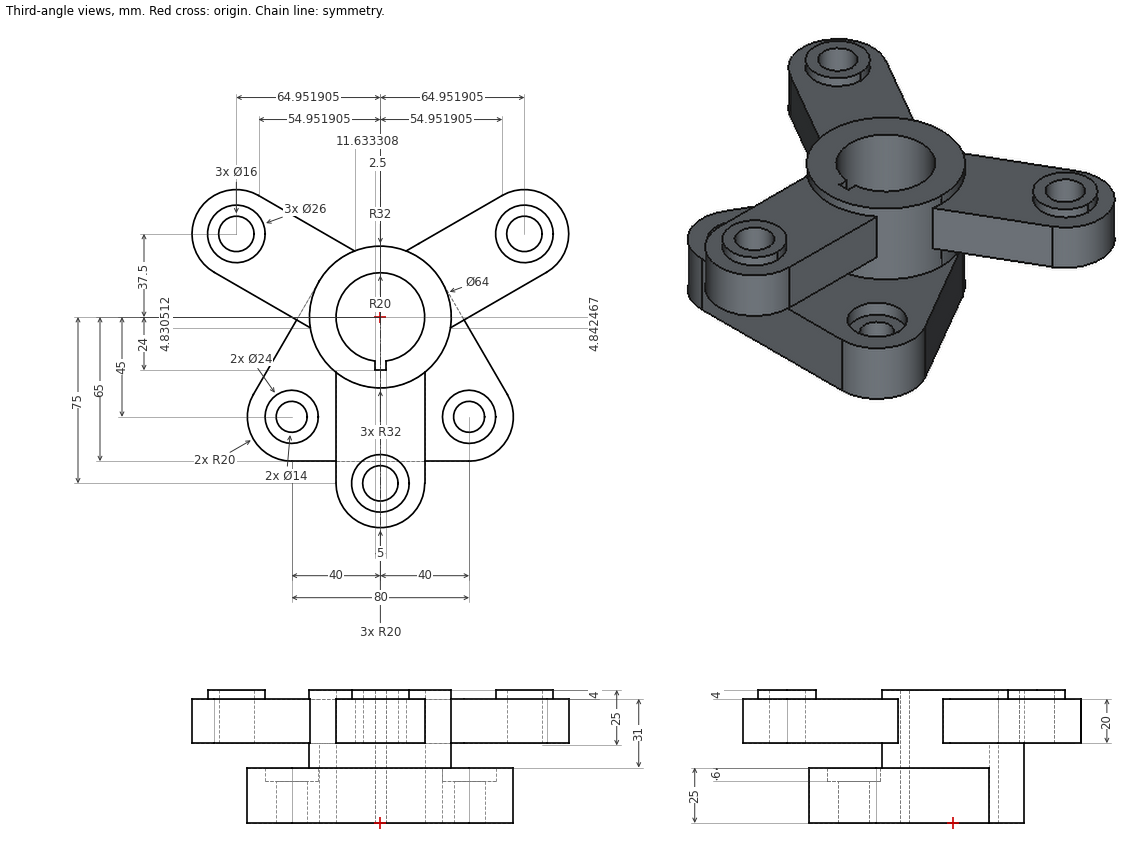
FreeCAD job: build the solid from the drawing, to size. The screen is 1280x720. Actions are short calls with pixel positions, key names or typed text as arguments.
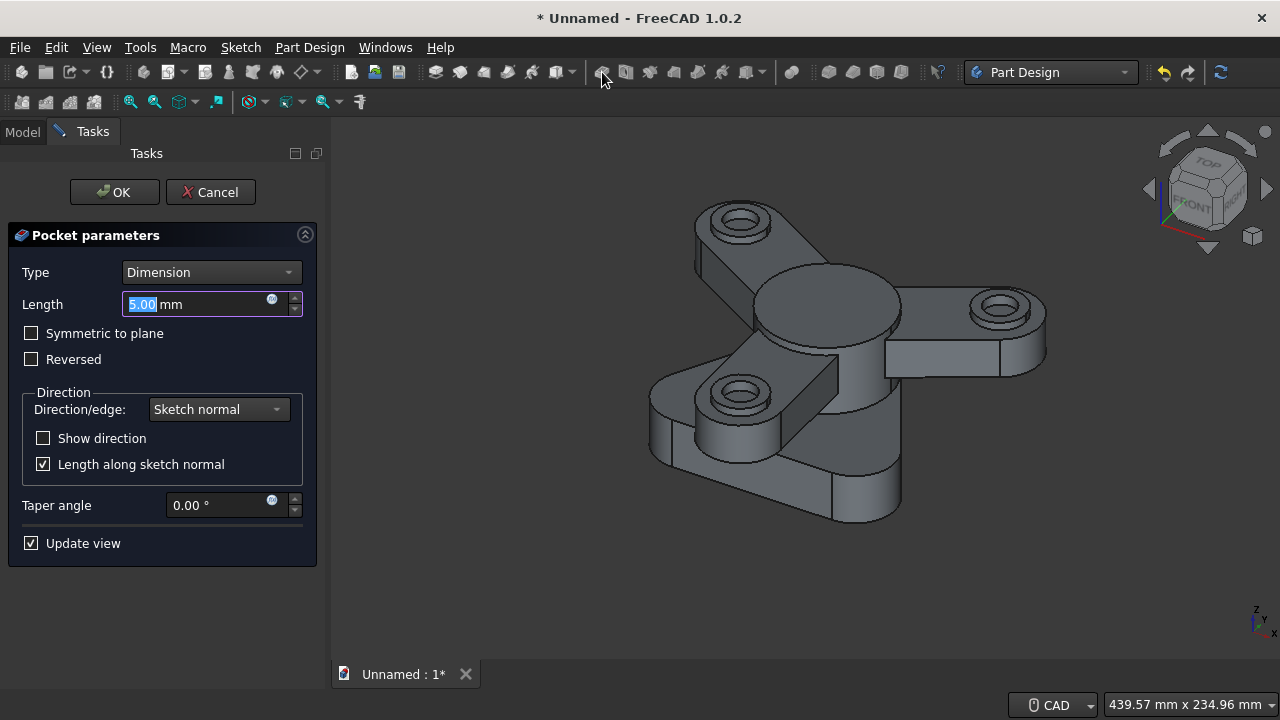
text(25)
key(Tab)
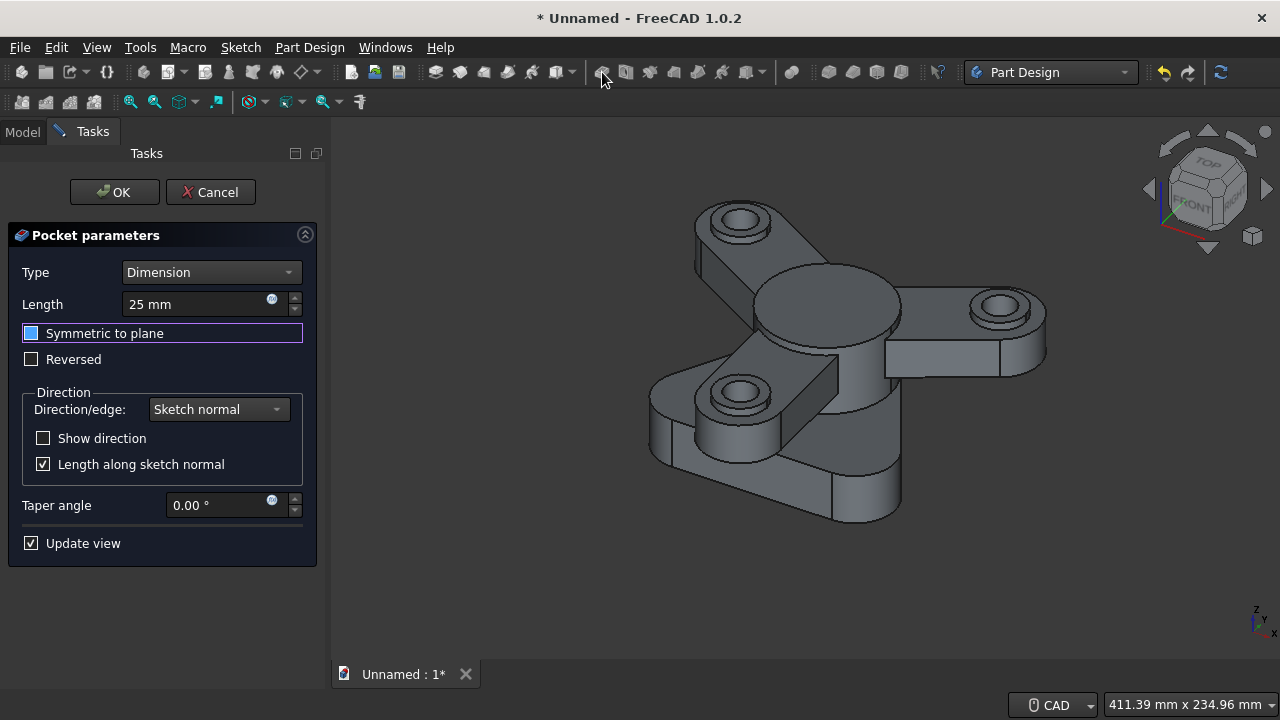
click(115, 192)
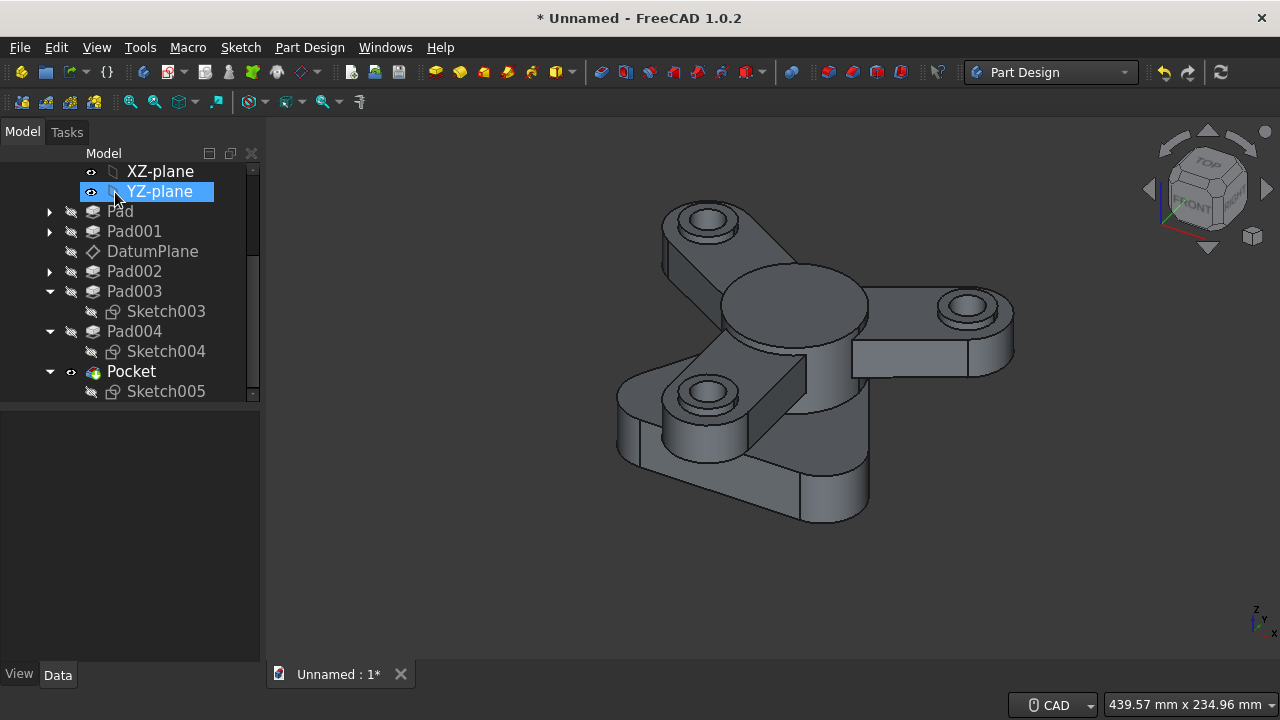
click(795, 305)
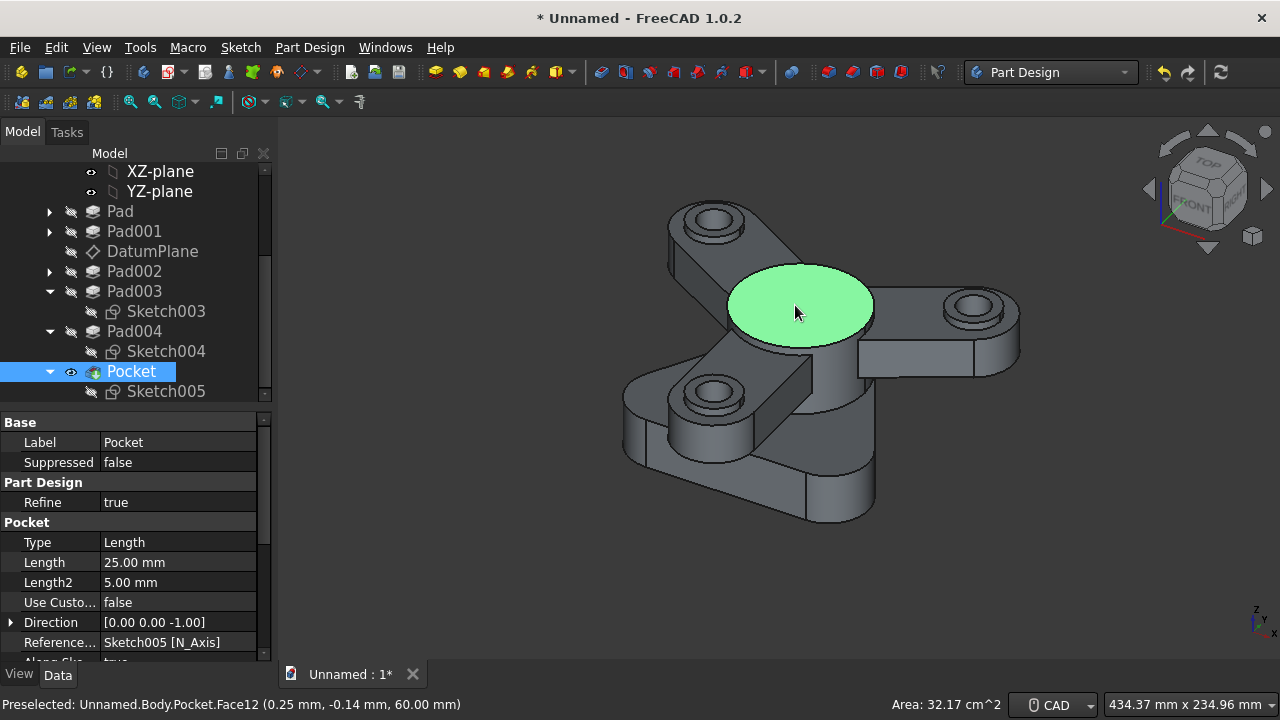
click(168, 72)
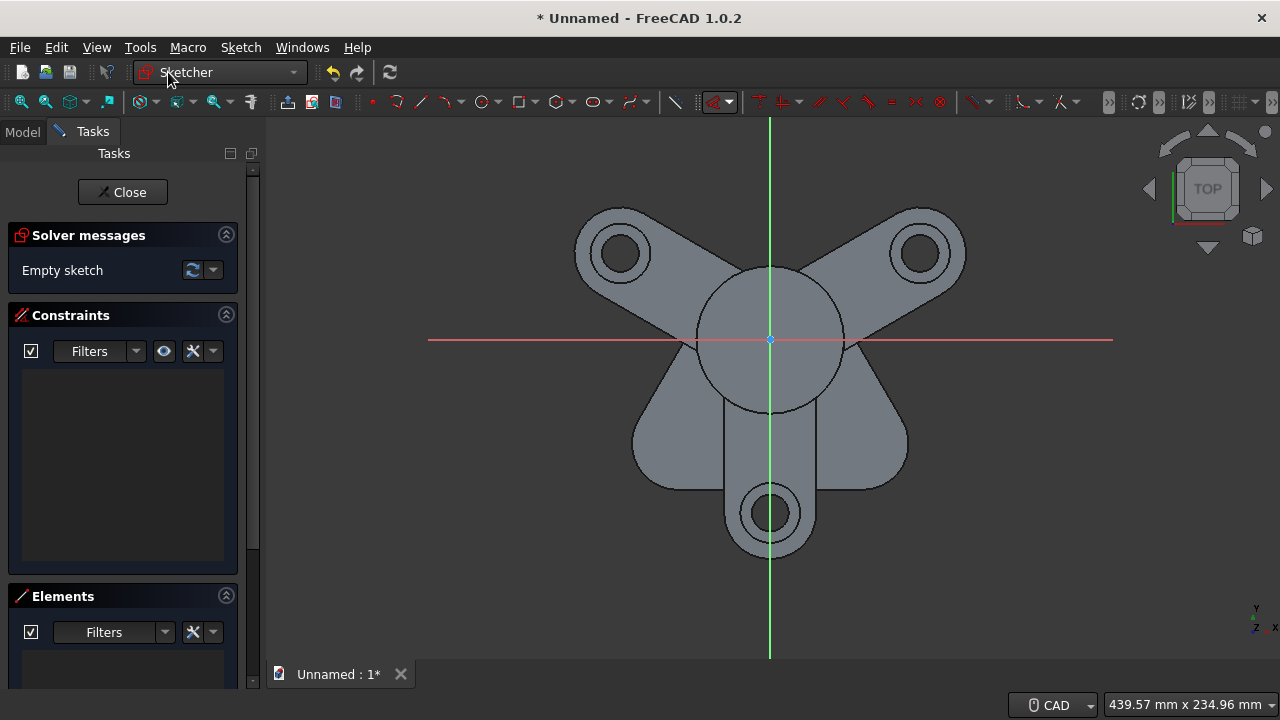
scroll(799, 326, up, 6)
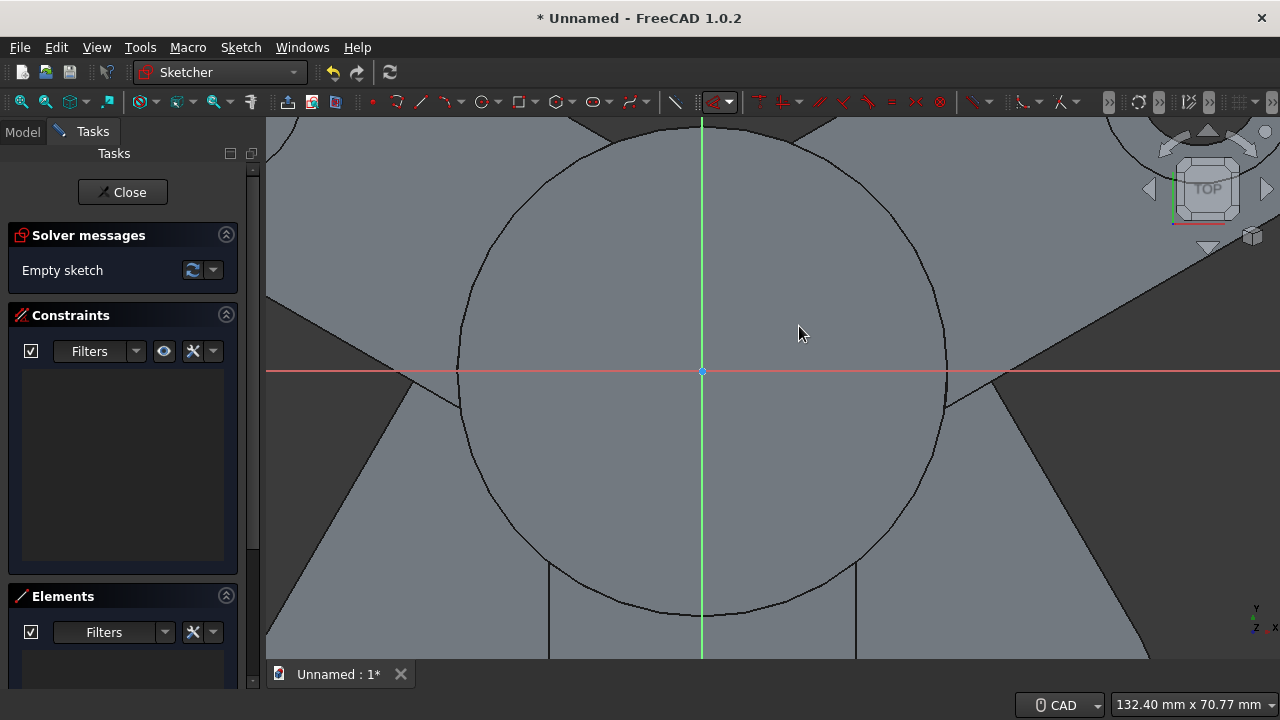
key(g)
key(m)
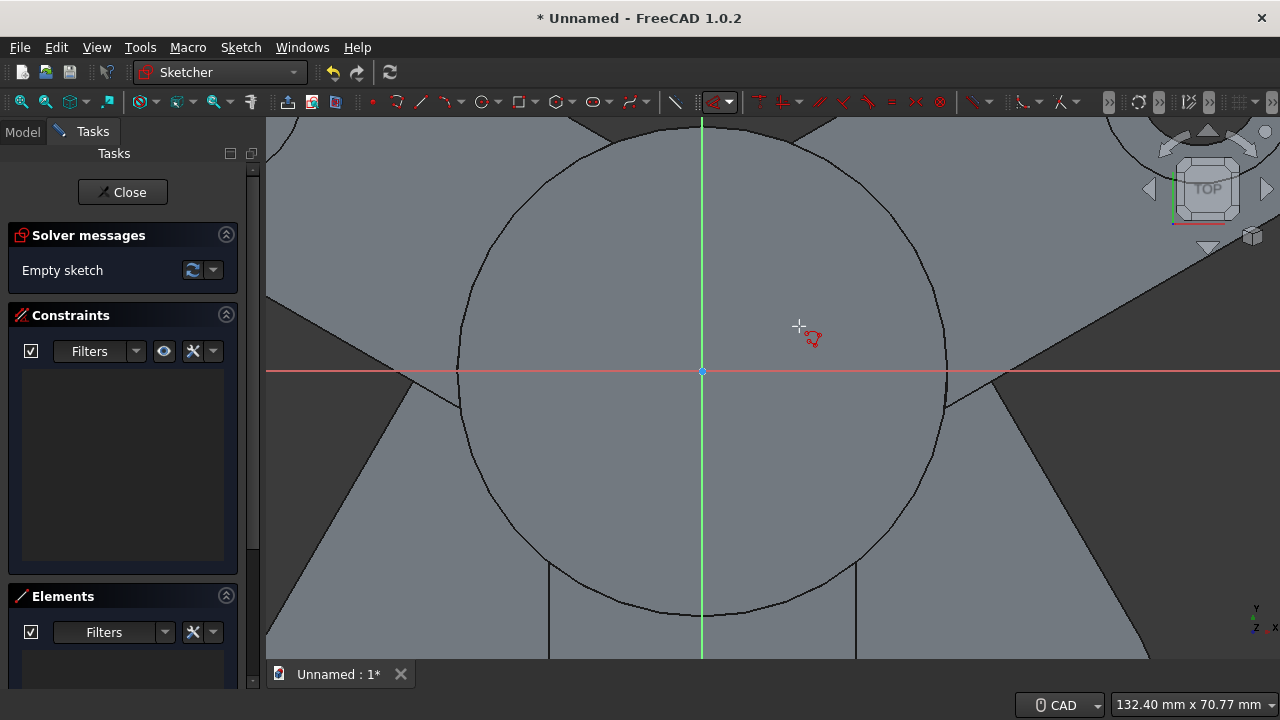
click(683, 523)
click(683, 555)
click(722, 555)
click(722, 523)
right_click(722, 523)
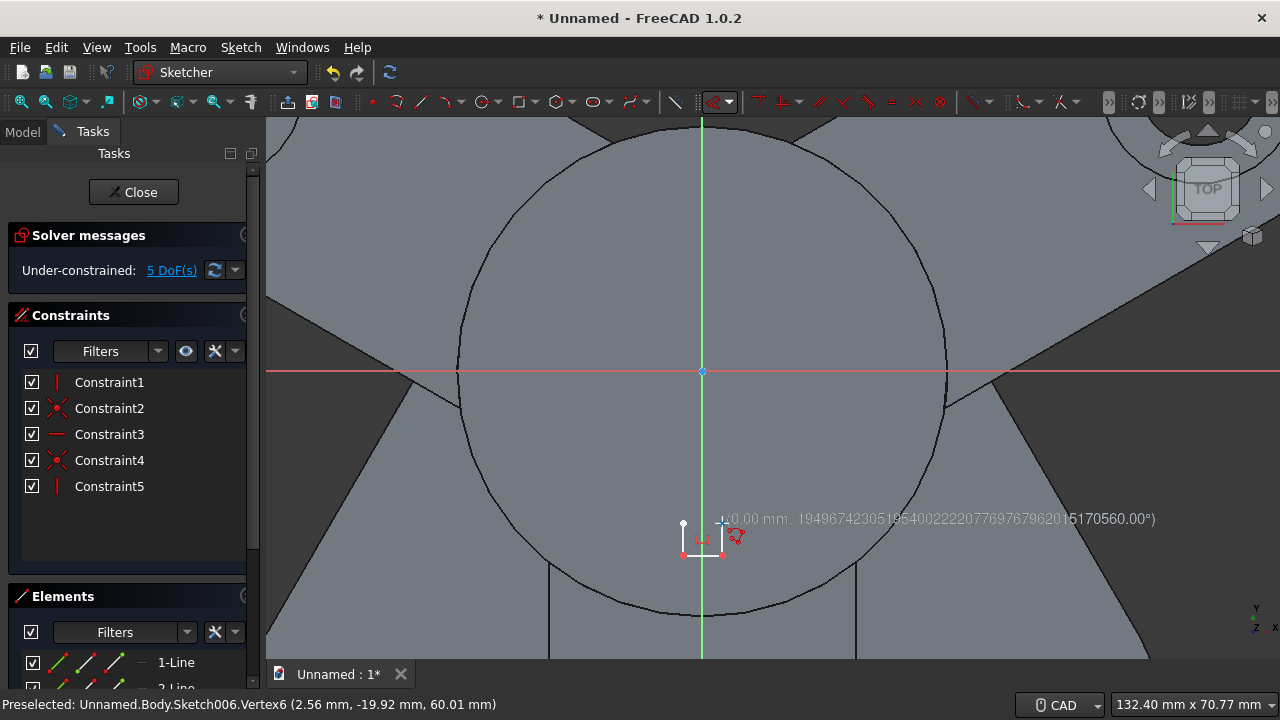
key(g)
key(3)
key(a)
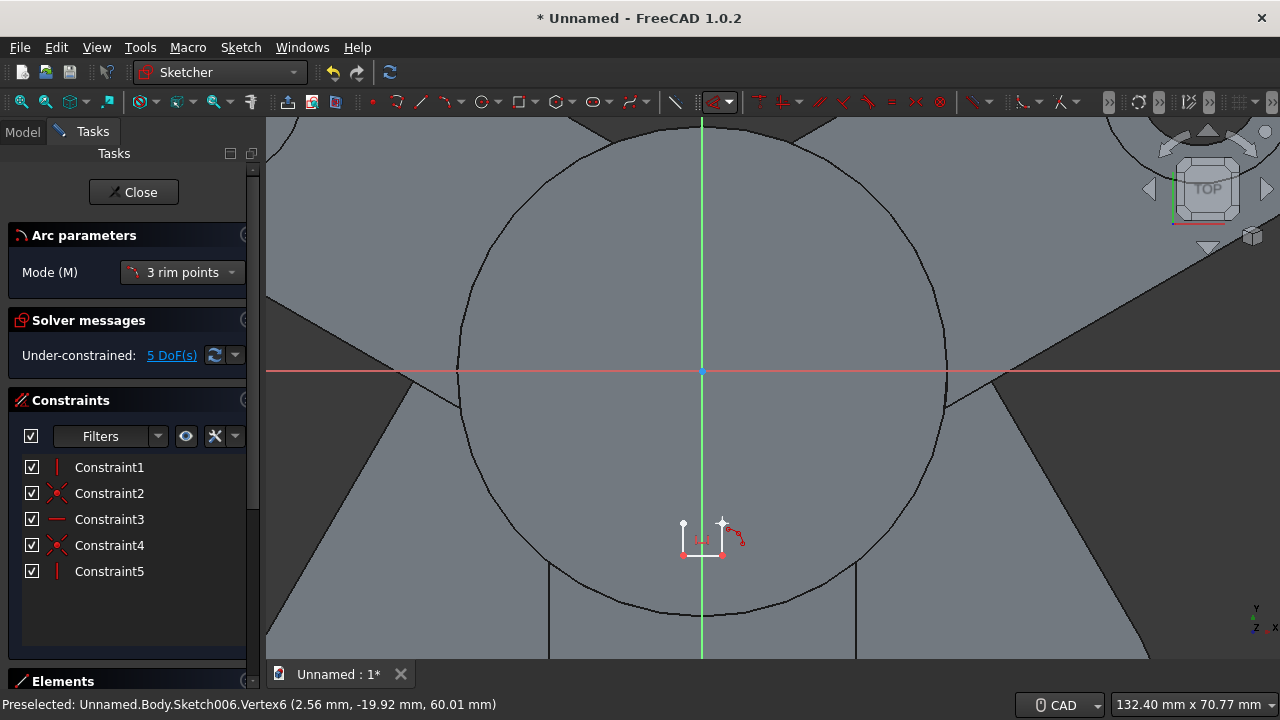
click(722, 524)
click(683, 524)
click(789, 245)
key(Escape)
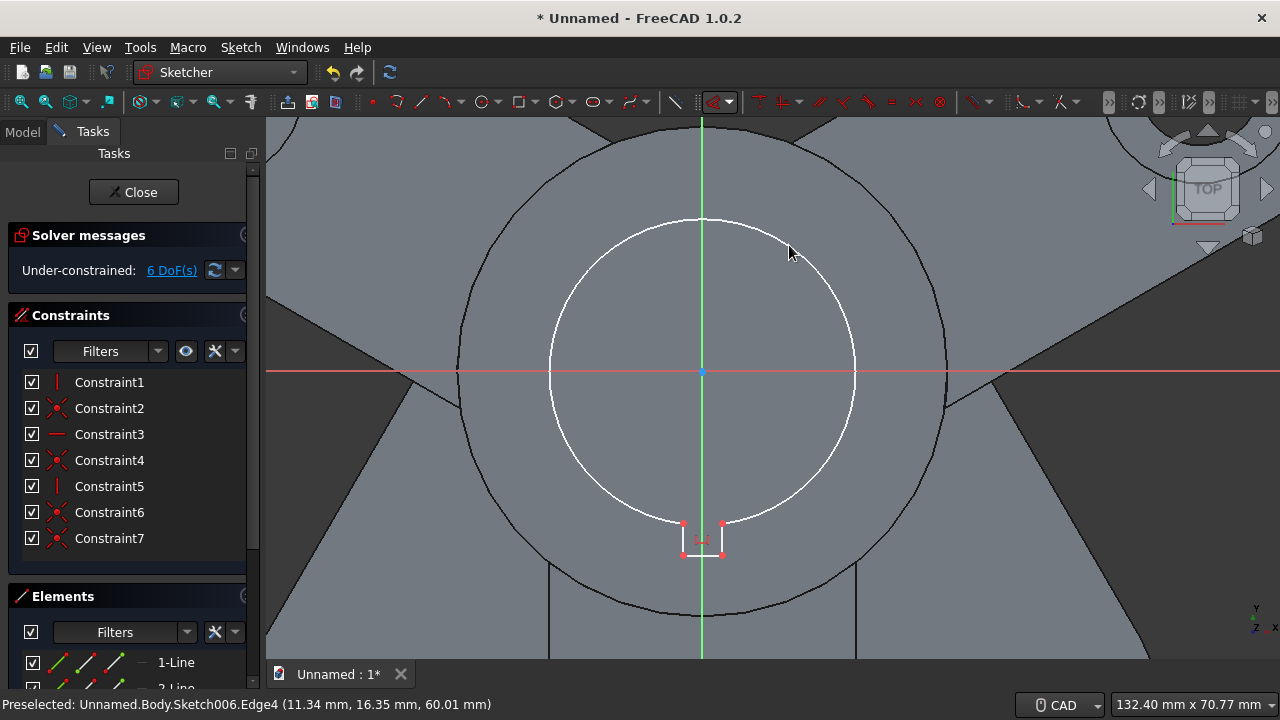
drag(692, 361, 713, 382)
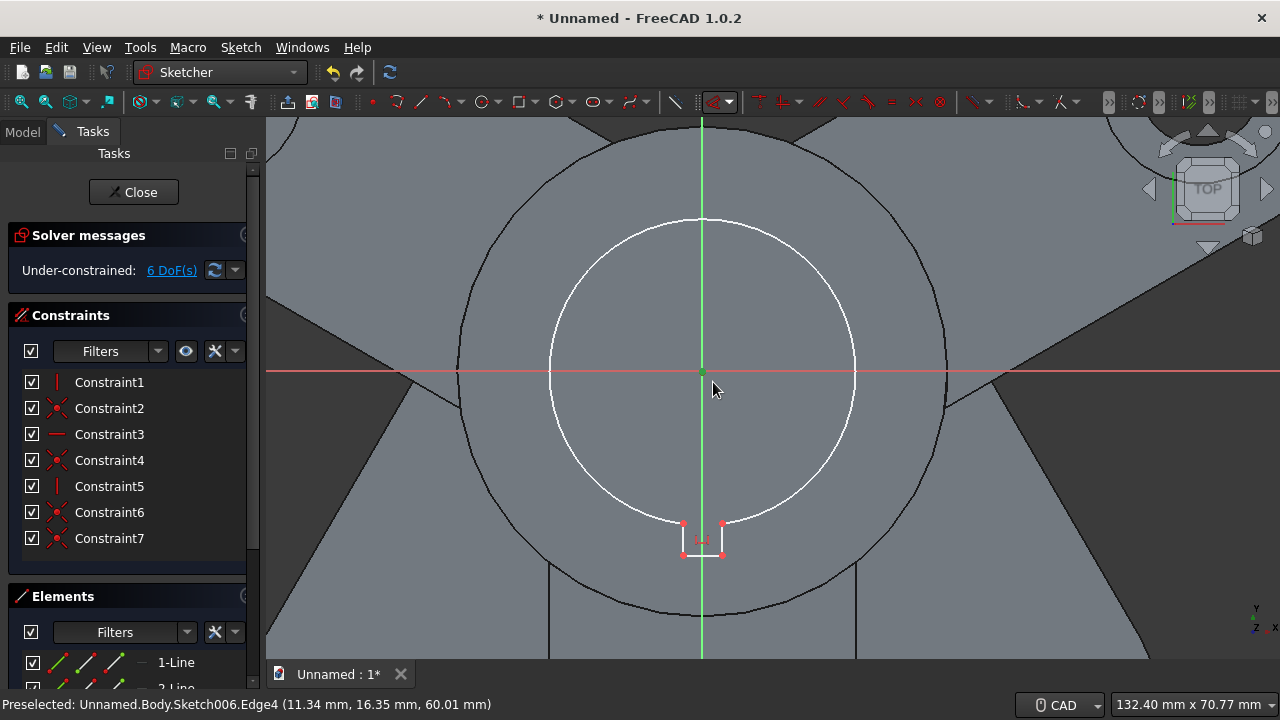
click(760, 102)